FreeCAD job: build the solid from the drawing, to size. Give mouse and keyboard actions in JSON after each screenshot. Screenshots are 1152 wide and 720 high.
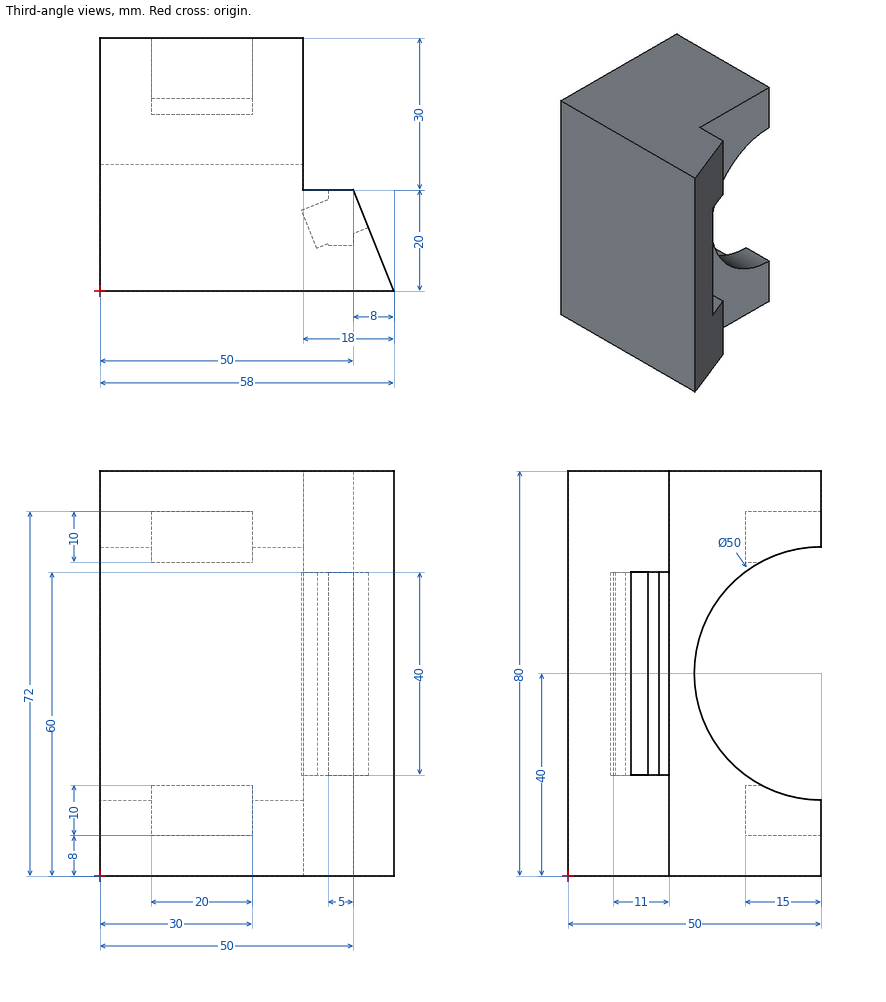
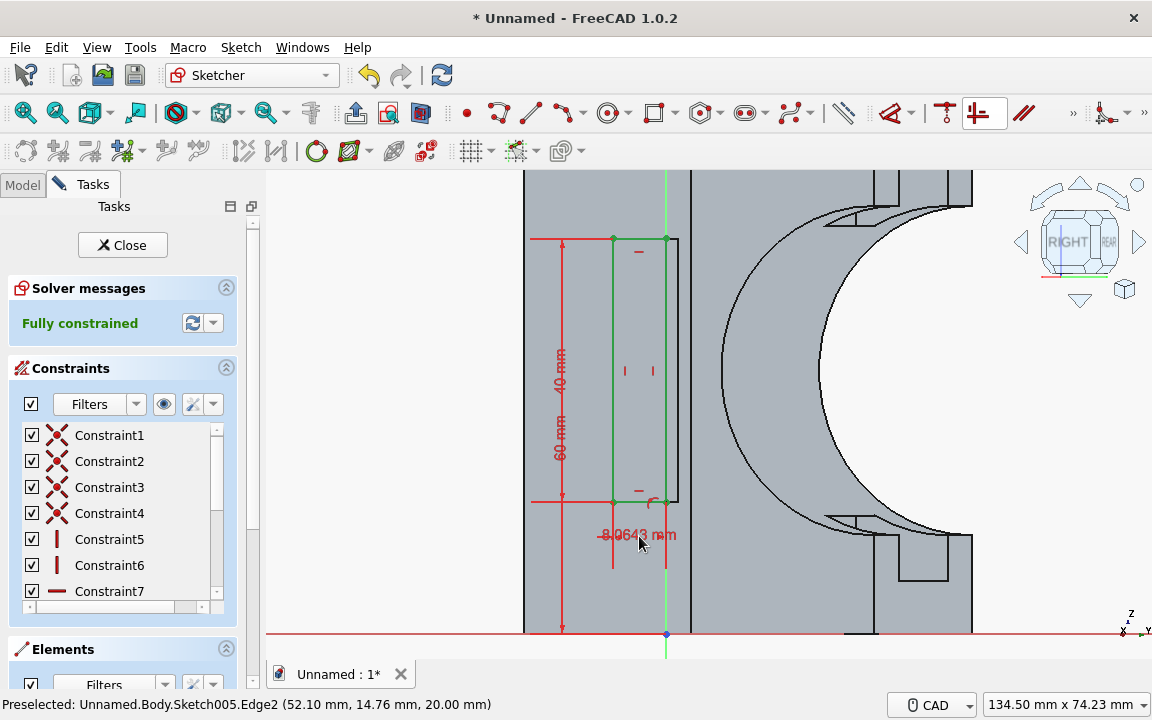
{"action": "left_click", "coordinate": [123, 245]}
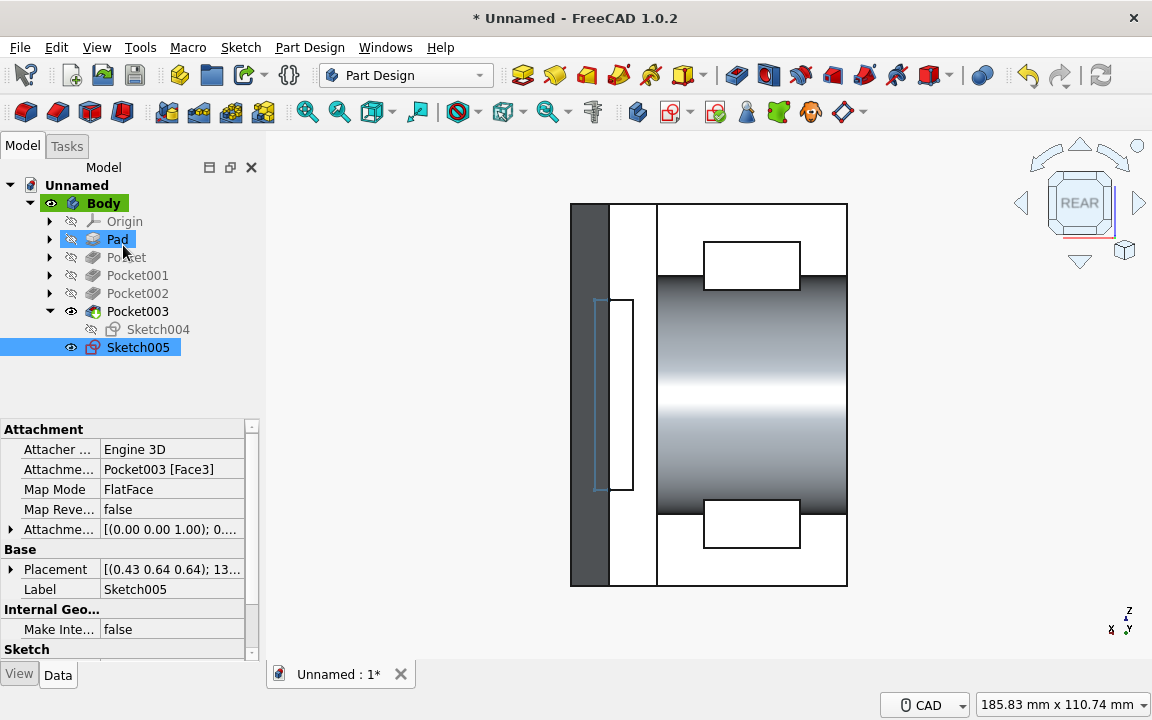
{"action": "left_click", "coordinate": [738, 76]}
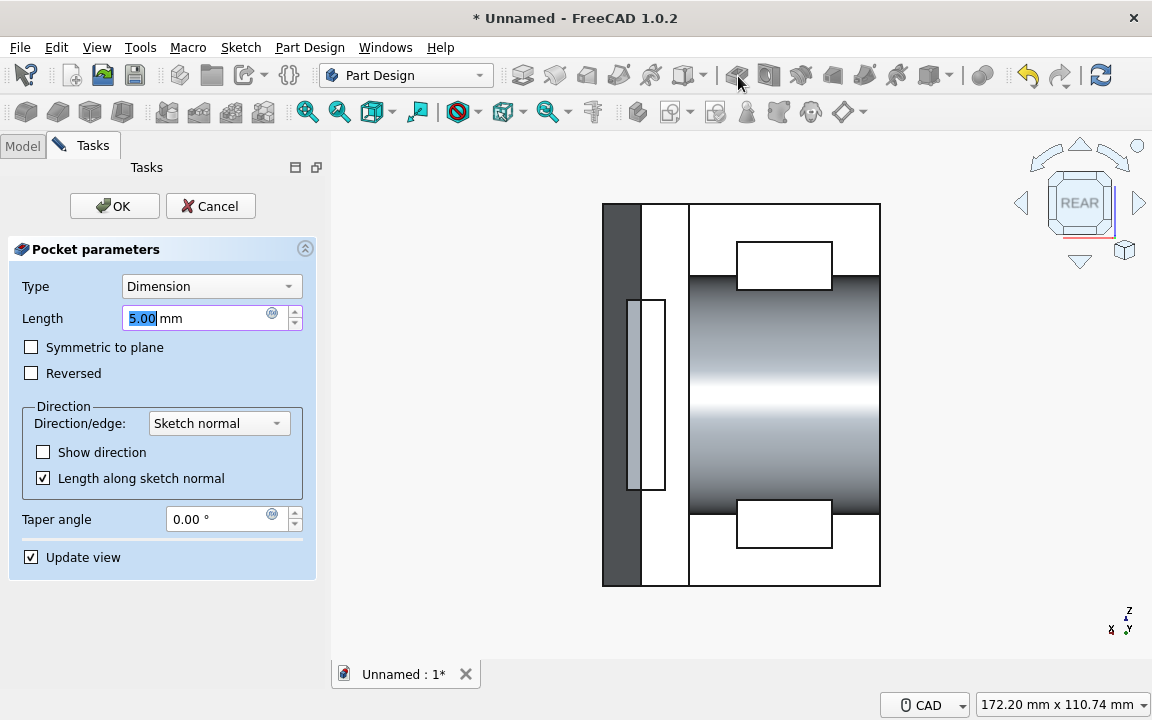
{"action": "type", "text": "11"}
{"action": "key", "text": "Tab"}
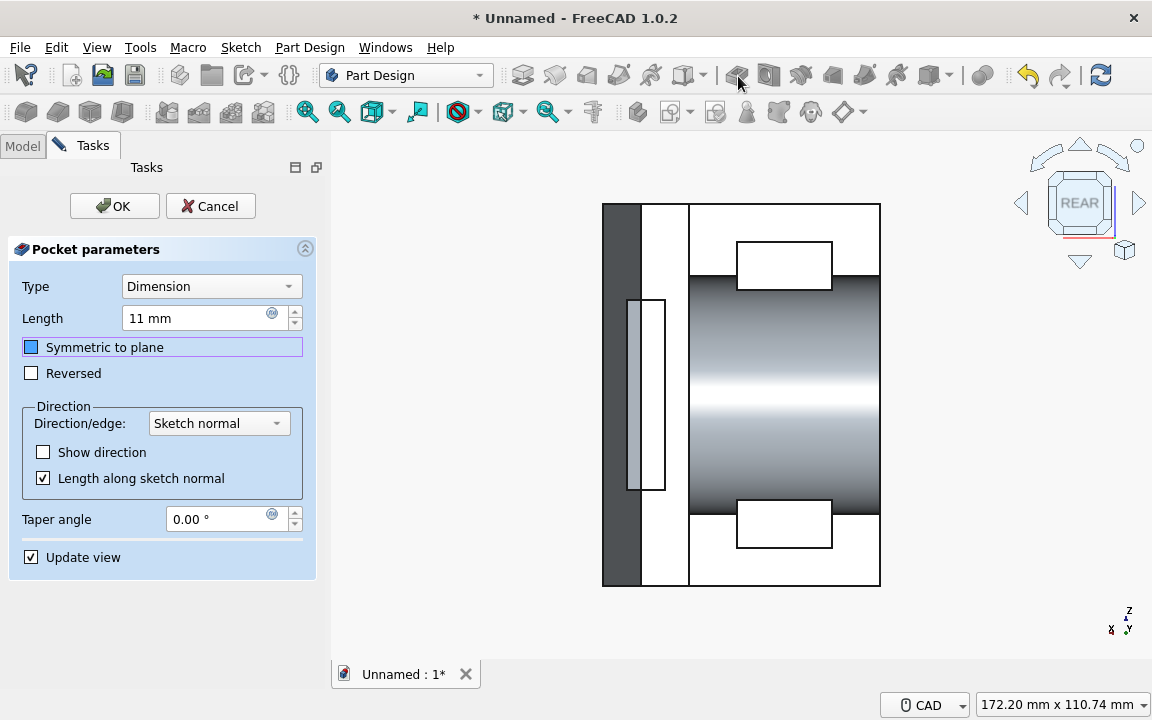
{"action": "left_click", "coordinate": [115, 206]}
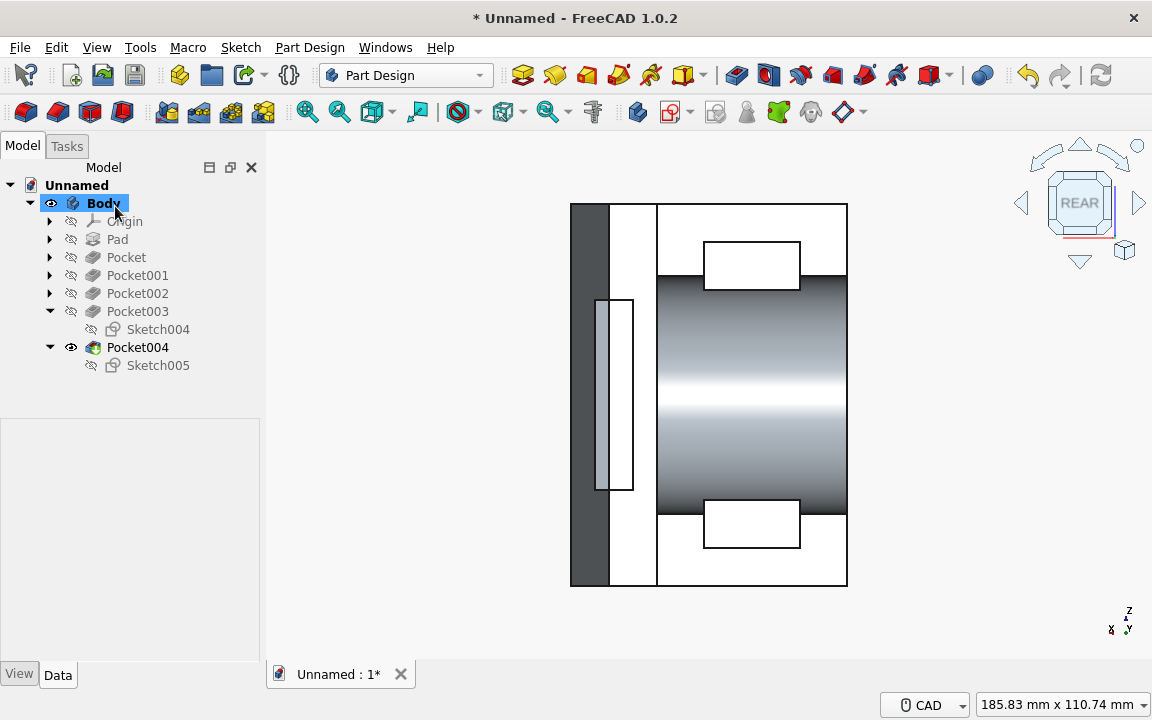
{"action": "key", "text": "0"}